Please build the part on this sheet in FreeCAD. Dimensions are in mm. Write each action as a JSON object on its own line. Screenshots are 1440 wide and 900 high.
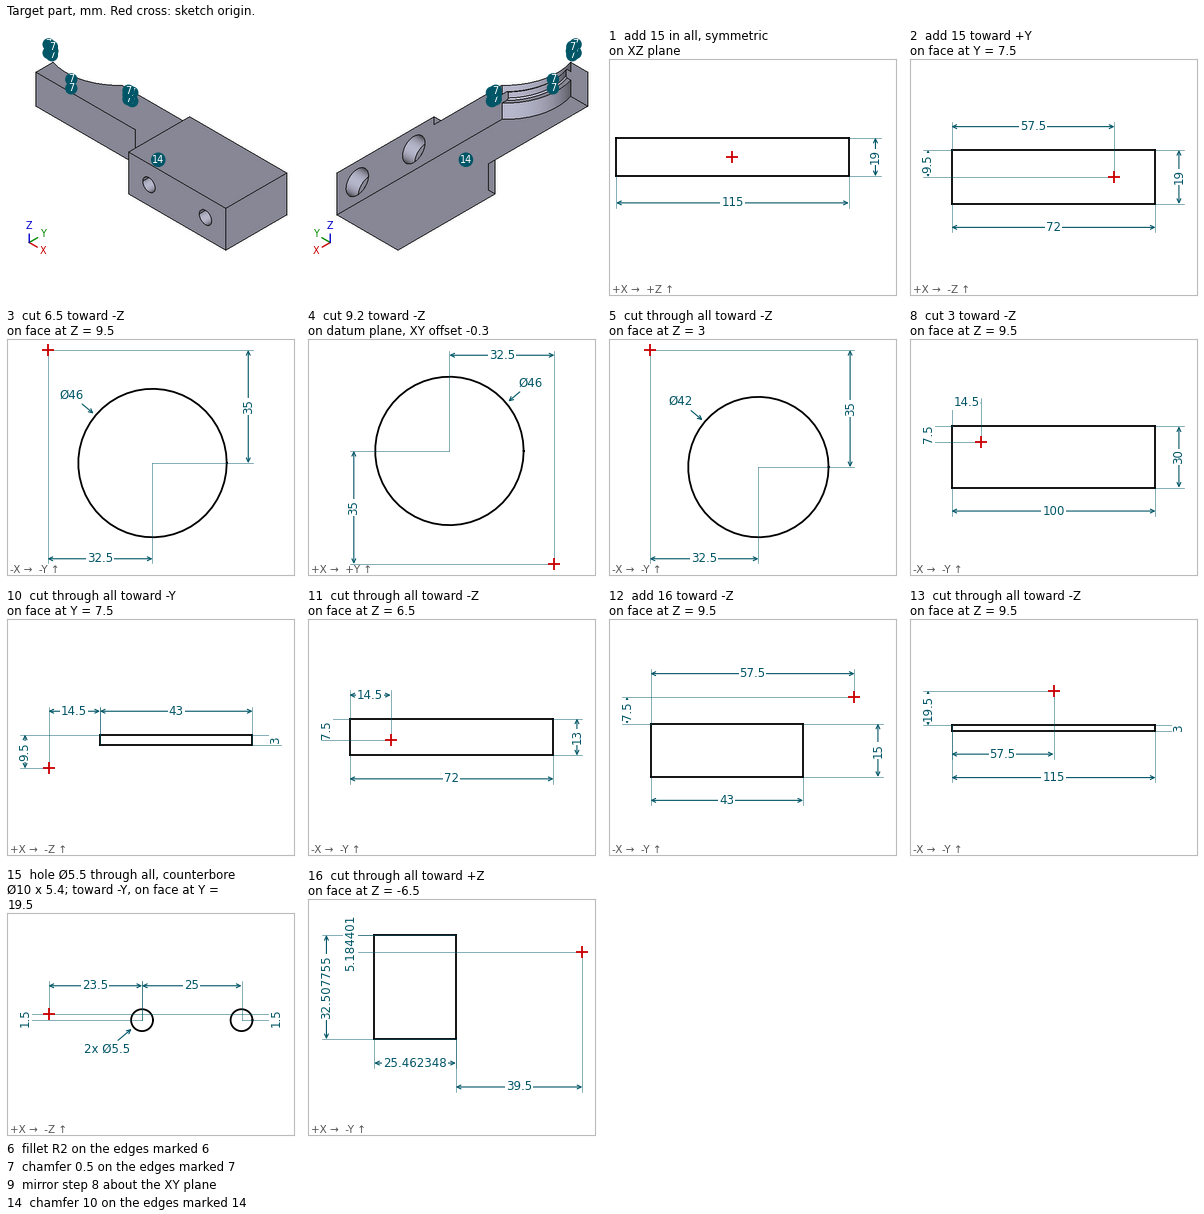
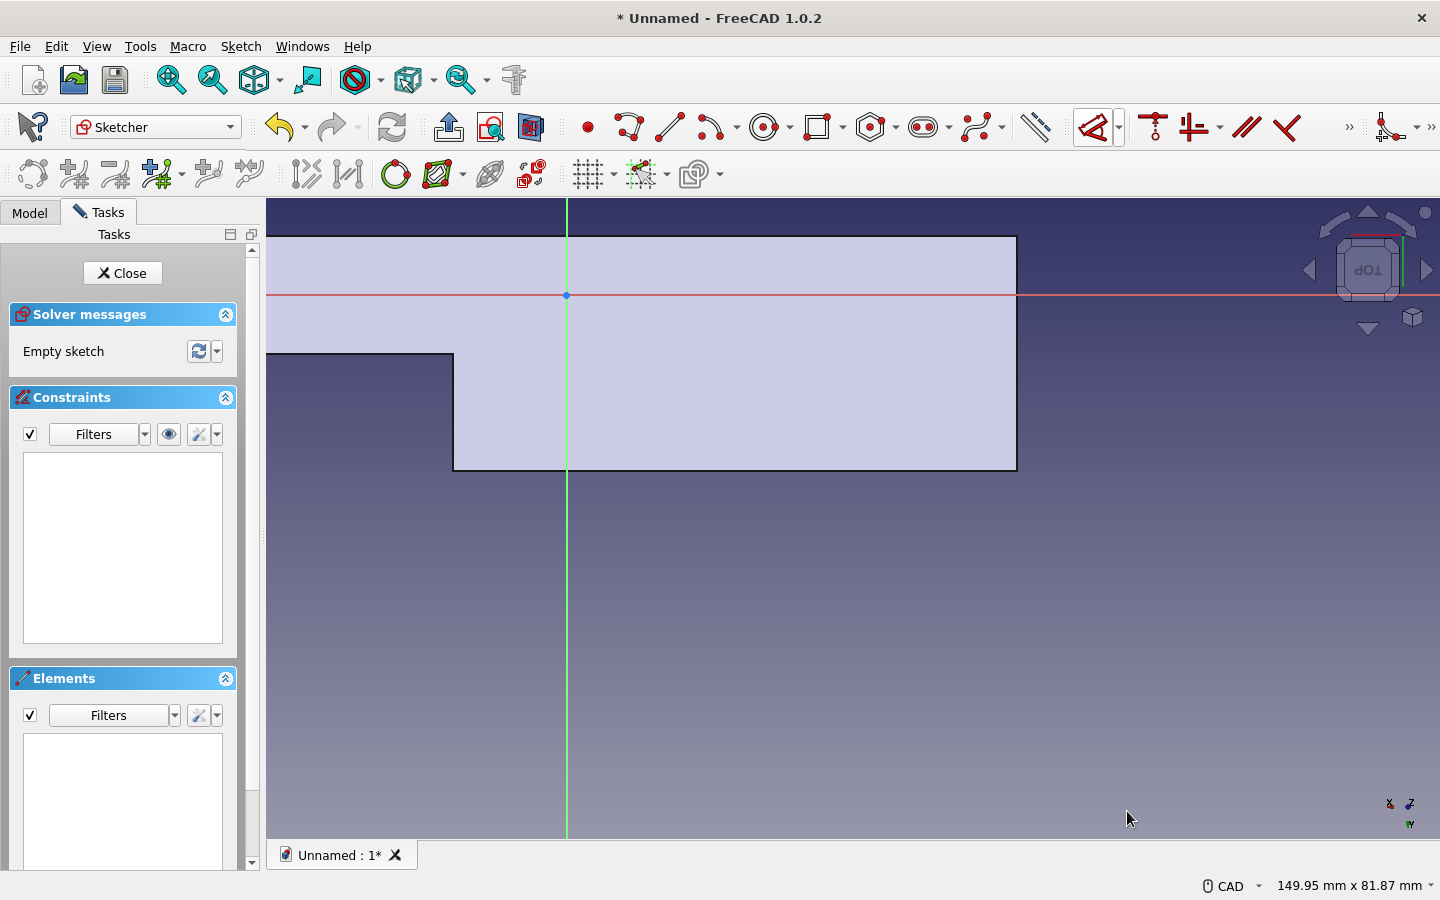
{"action": "left_click", "coordinate": [764, 128]}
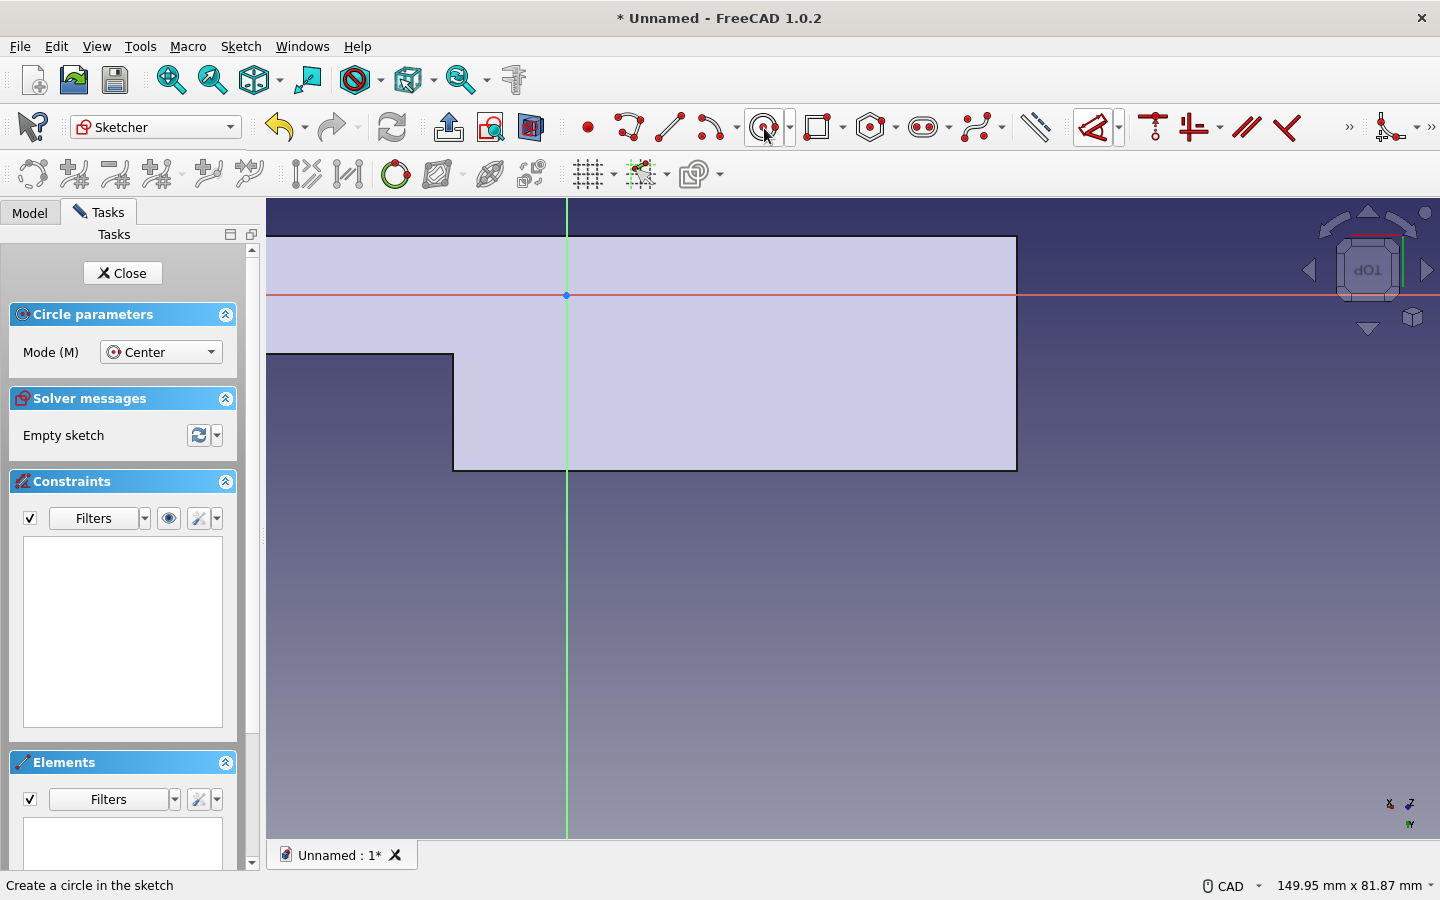
{"action": "left_click", "coordinate": [821, 569]}
{"action": "mouse_move", "coordinate": [948, 442]}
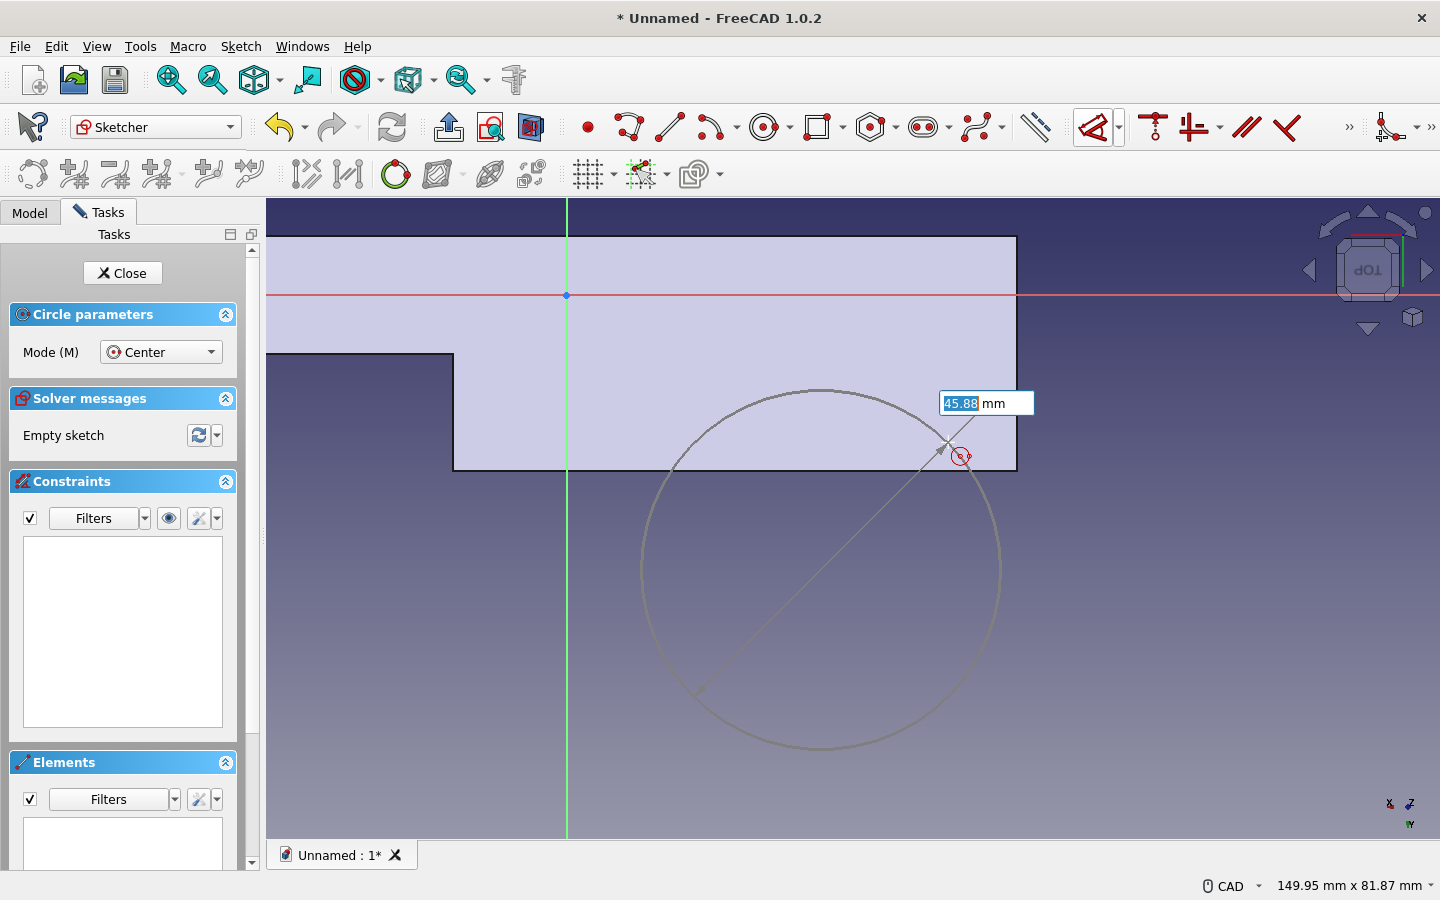
{"action": "type", "text": "46"}
{"action": "key", "text": "Return"}
{"action": "key", "text": "Escape"}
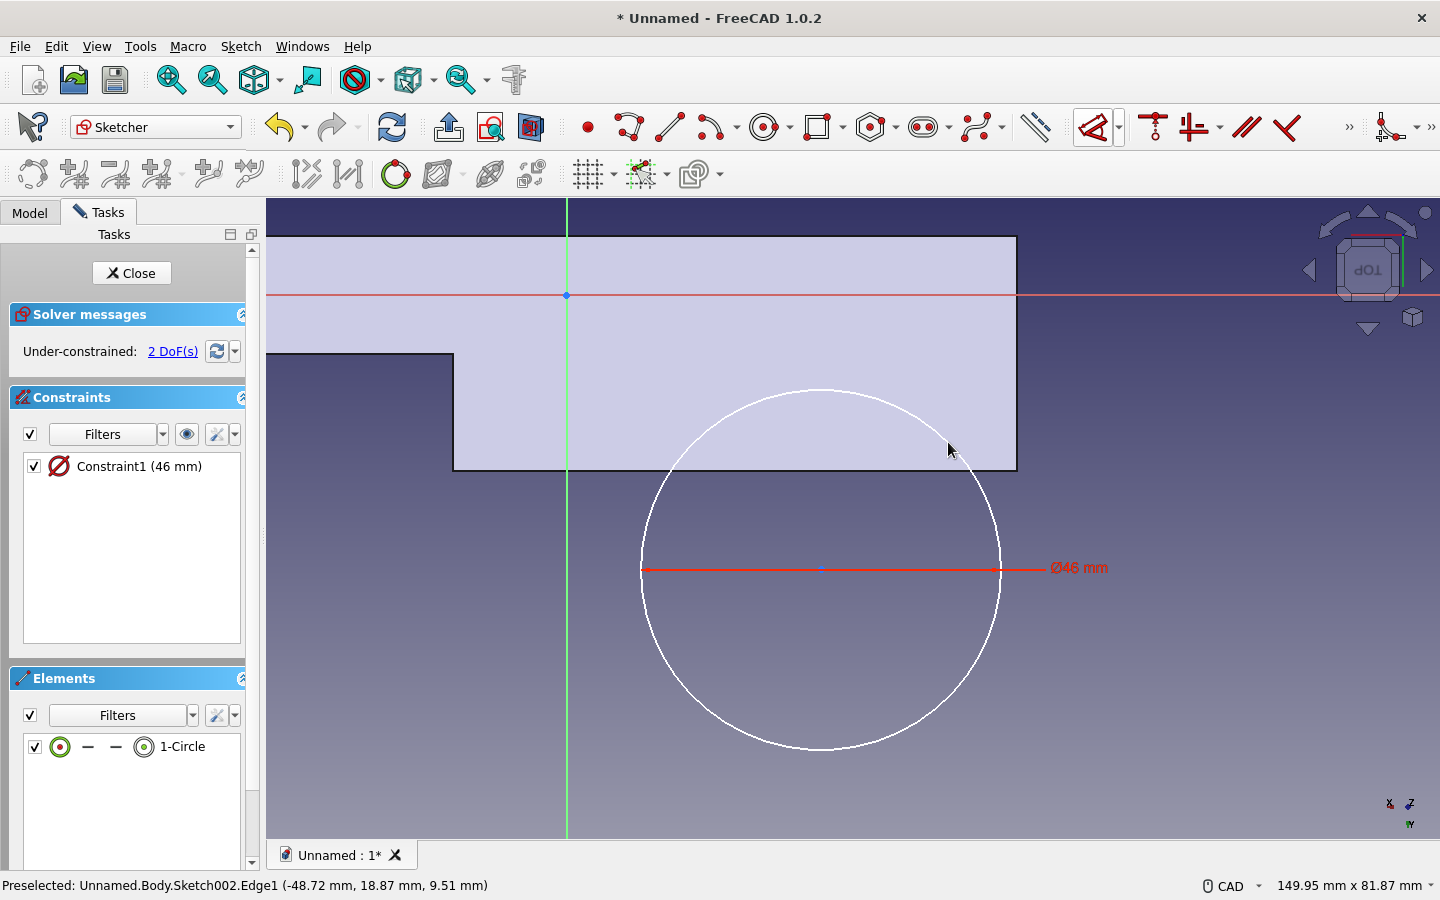
{"action": "left_click", "coordinate": [821, 570]}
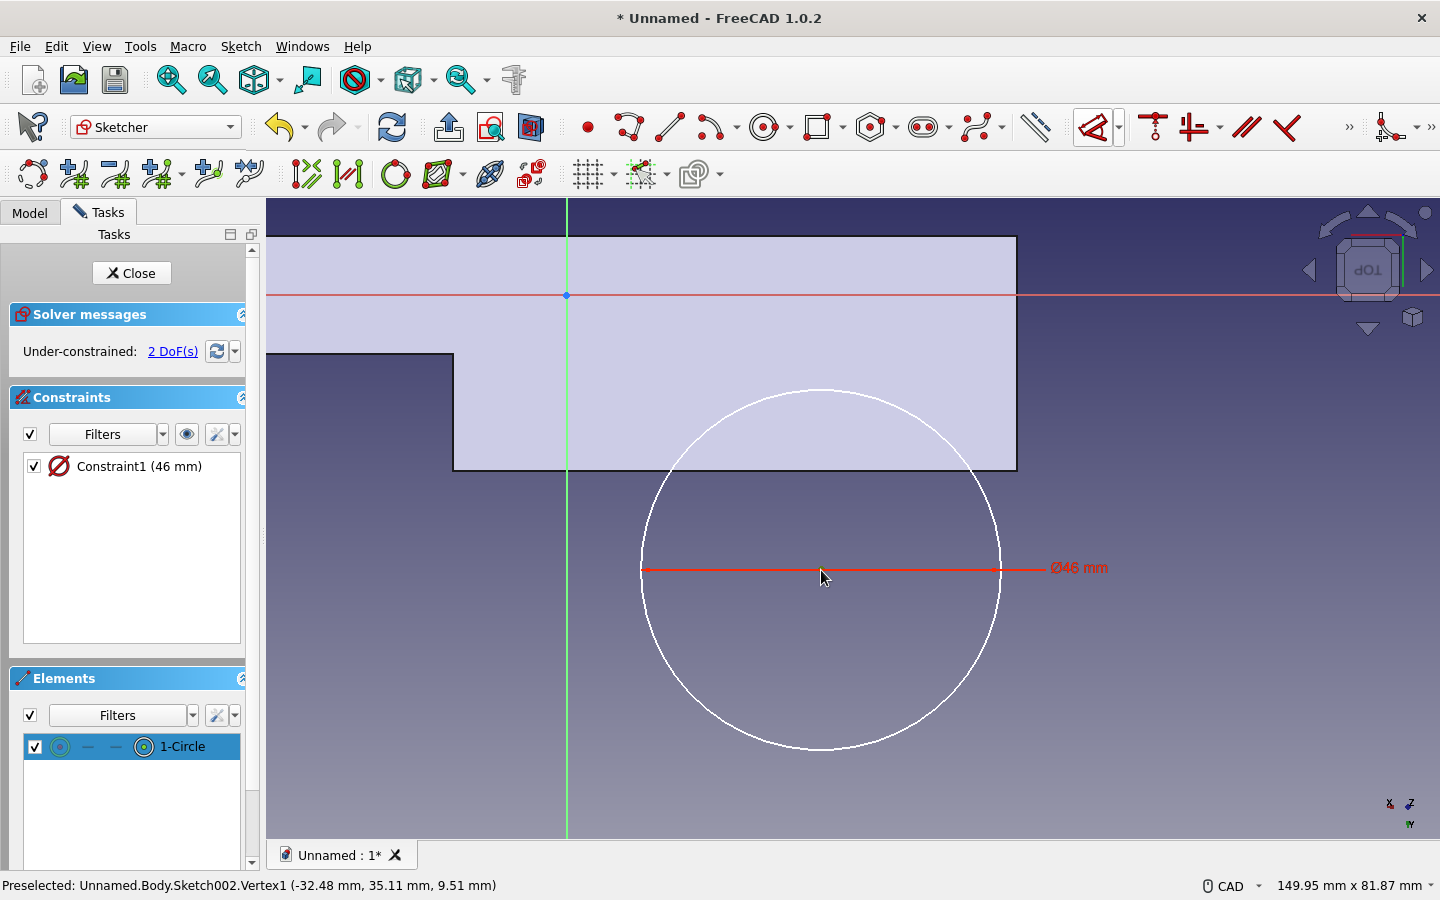
{"action": "left_click", "coordinate": [1118, 128]}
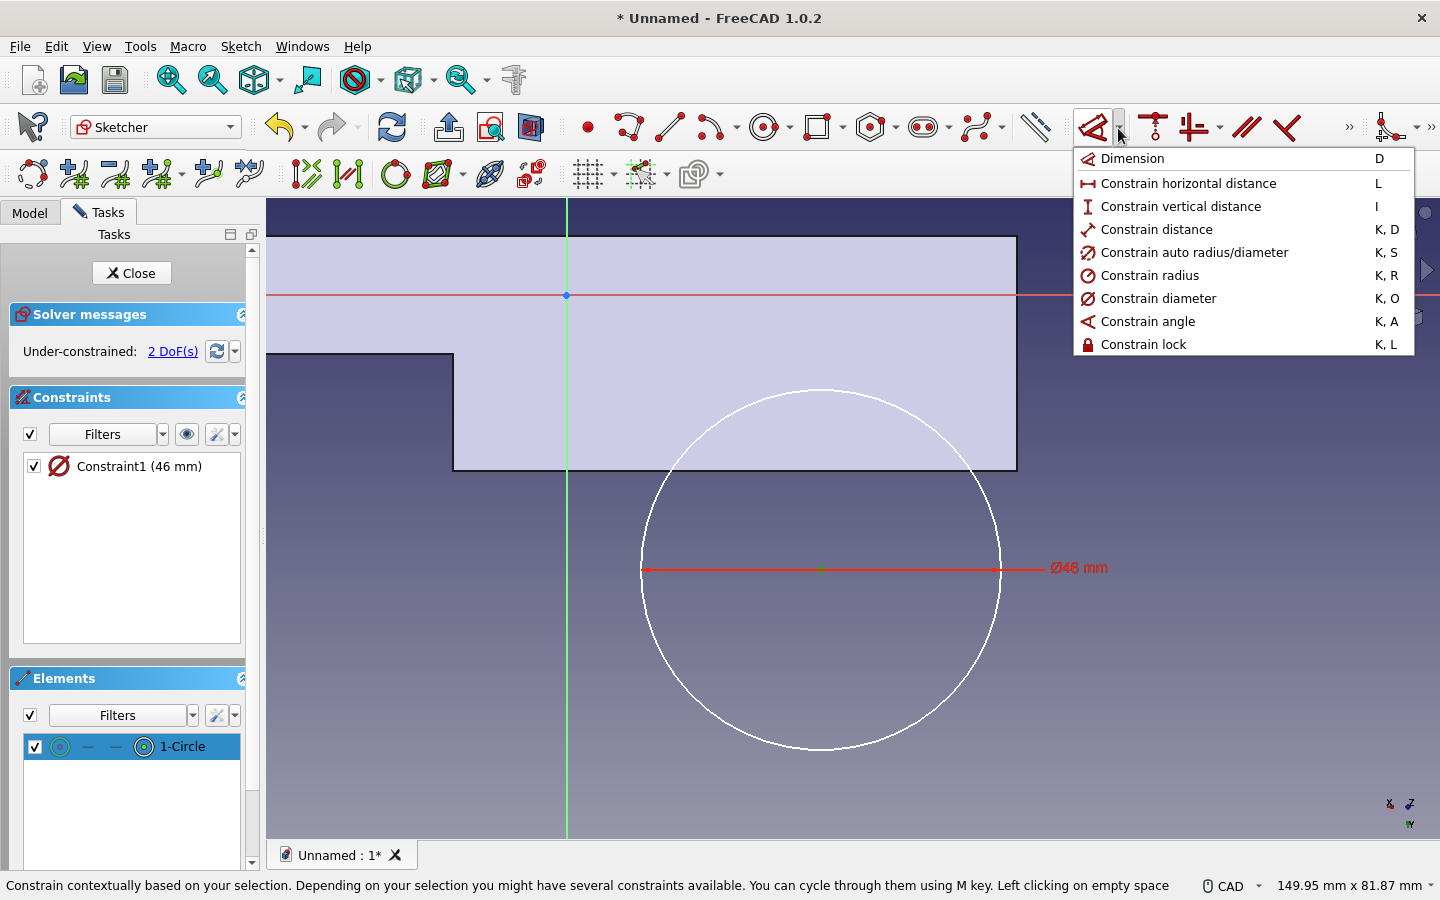
{"action": "left_click", "coordinate": [1244, 206]}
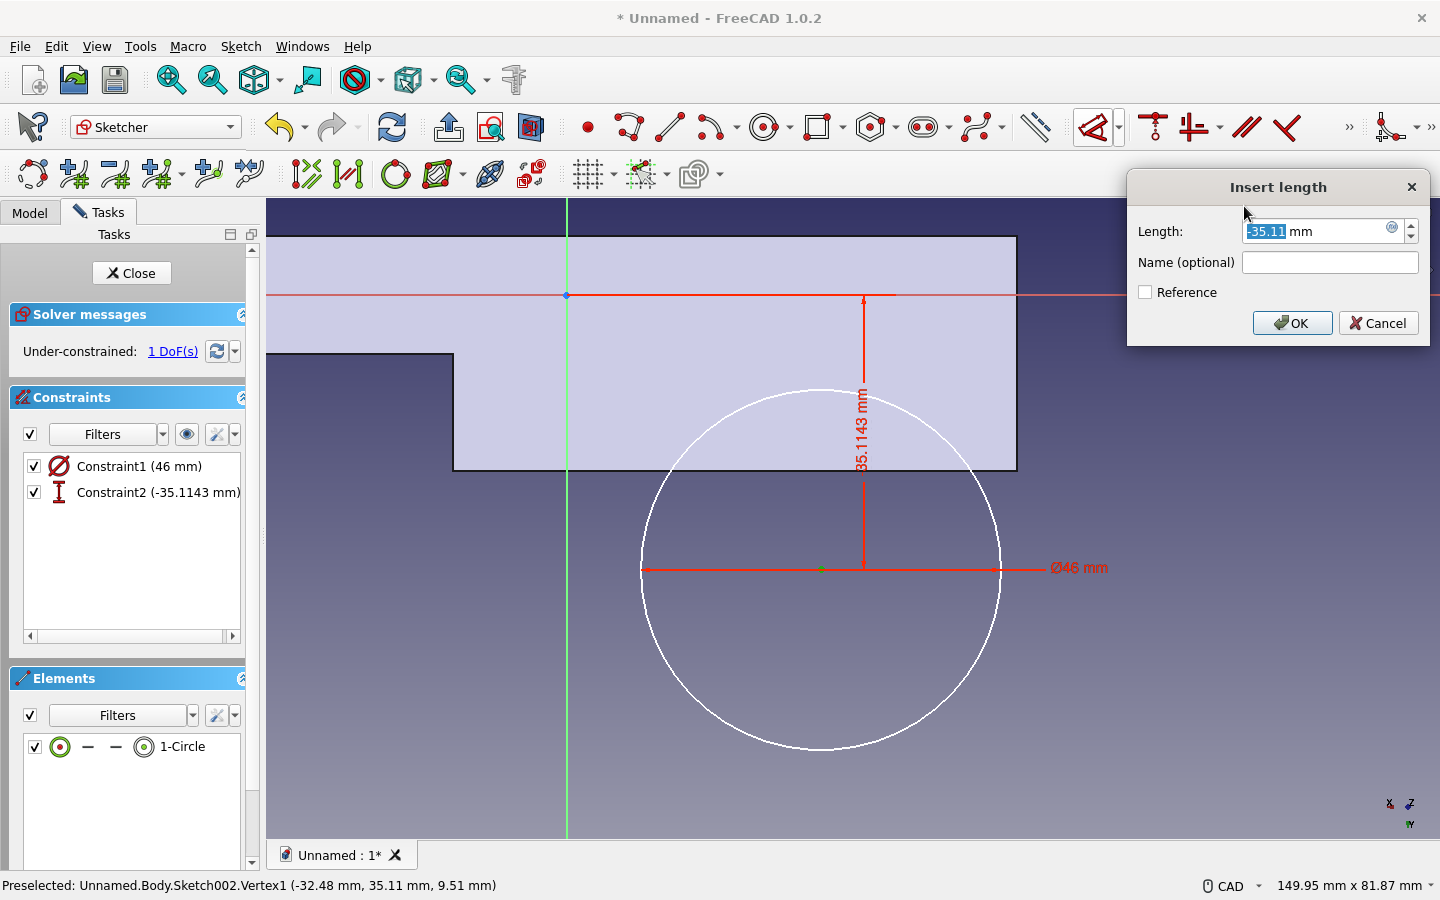
{"action": "type", "text": "-35"}
{"action": "key", "text": "Return"}